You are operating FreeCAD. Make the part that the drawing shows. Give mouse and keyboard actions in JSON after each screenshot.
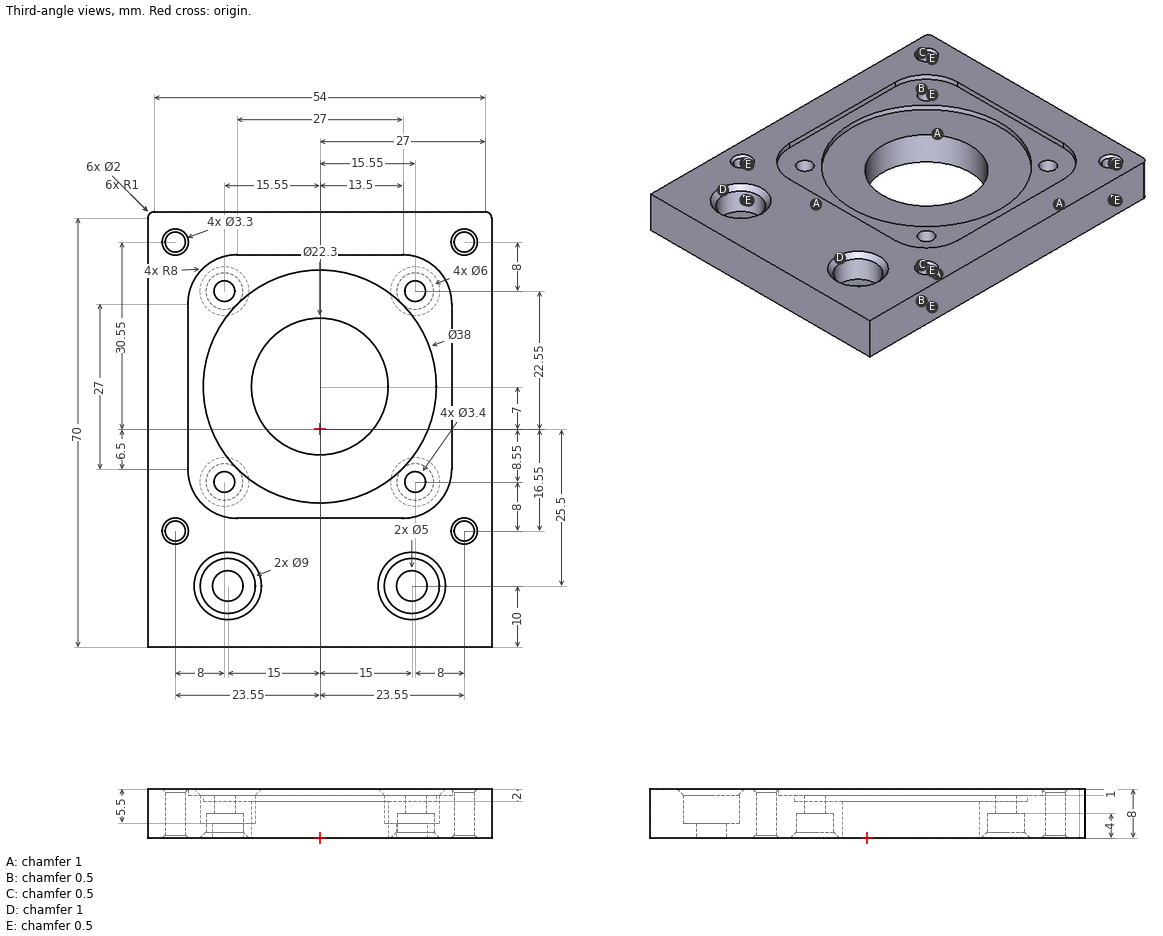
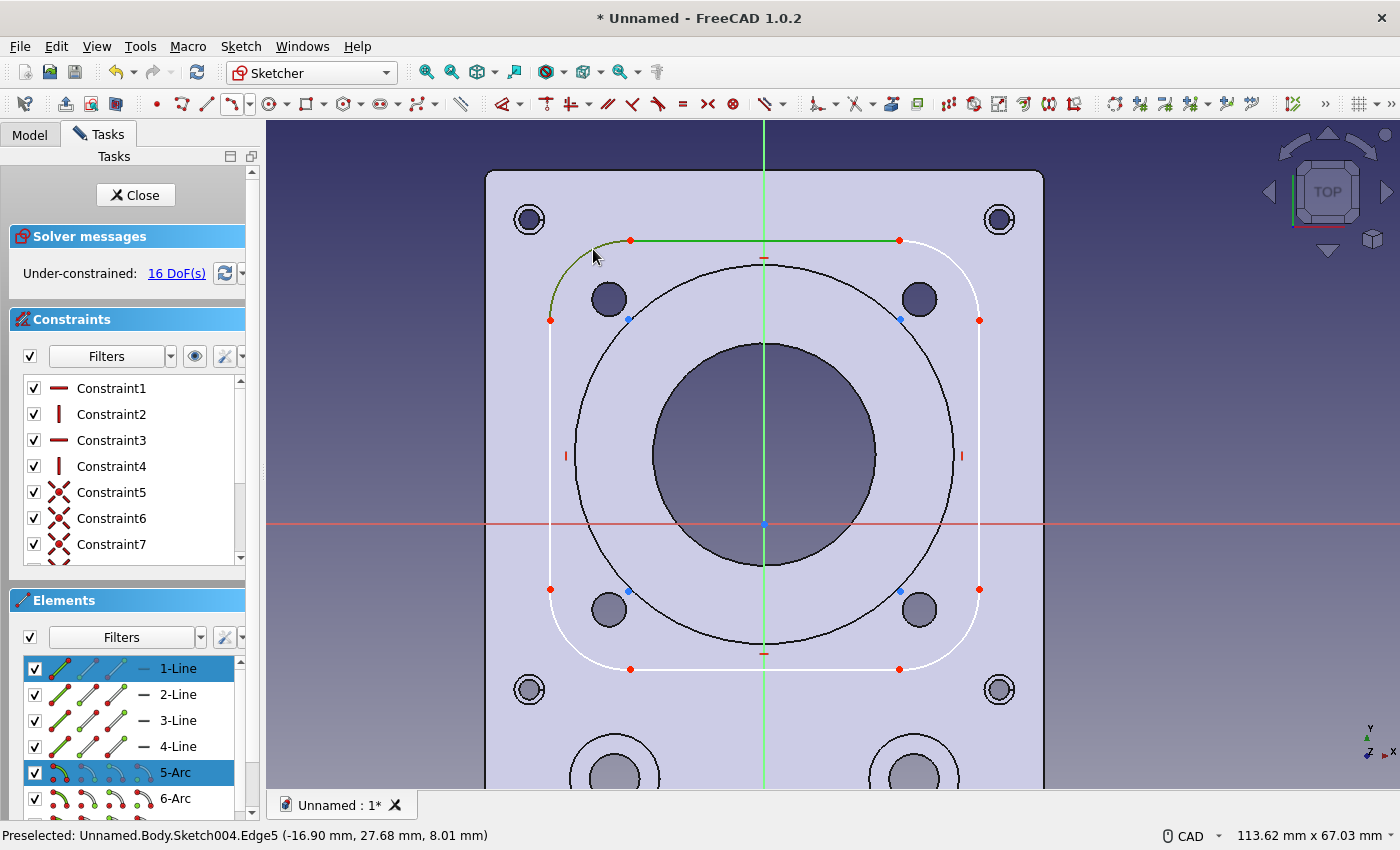
{"action": "key", "text": "t"}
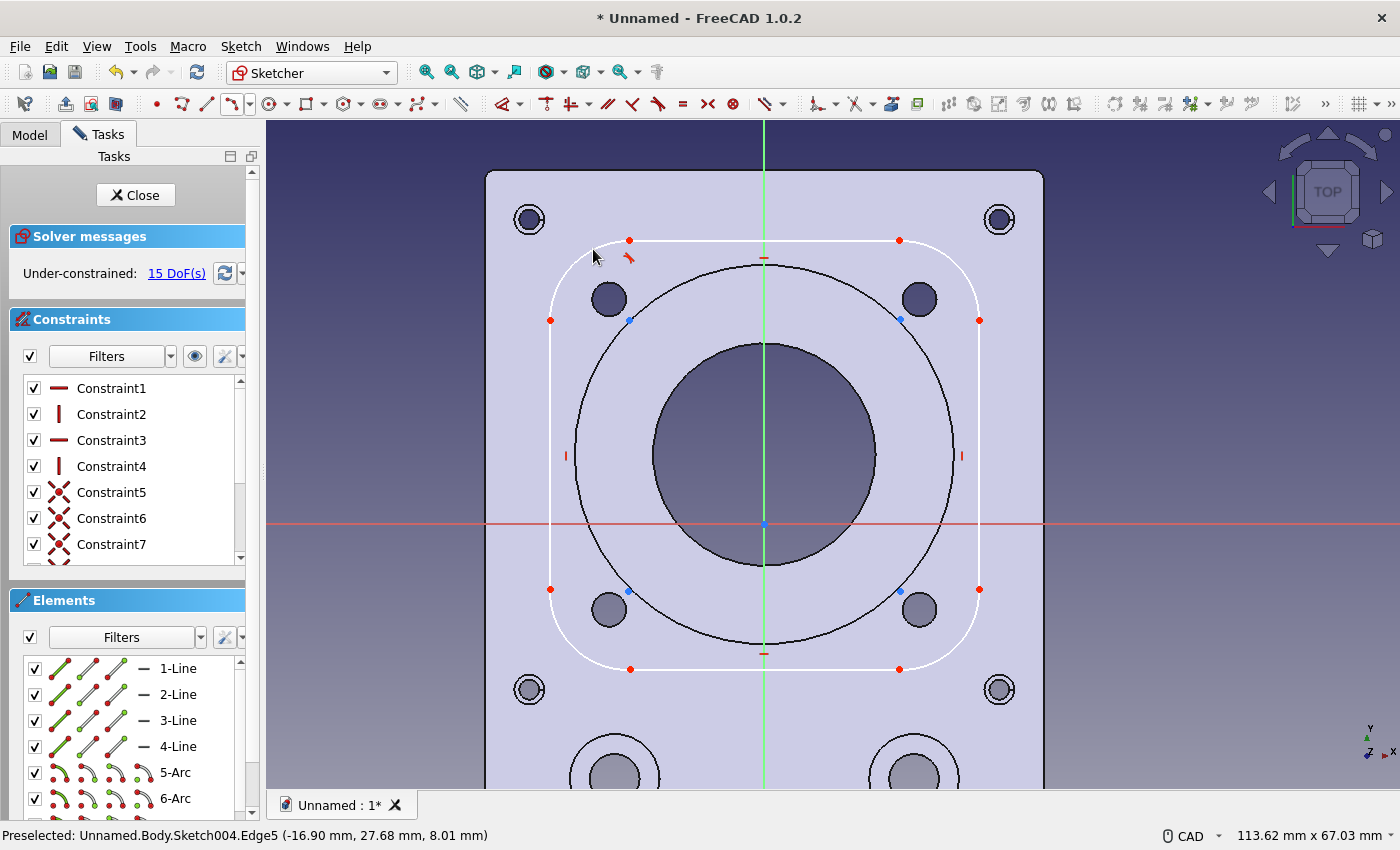
{"action": "left_click", "coordinate": [818, 241]}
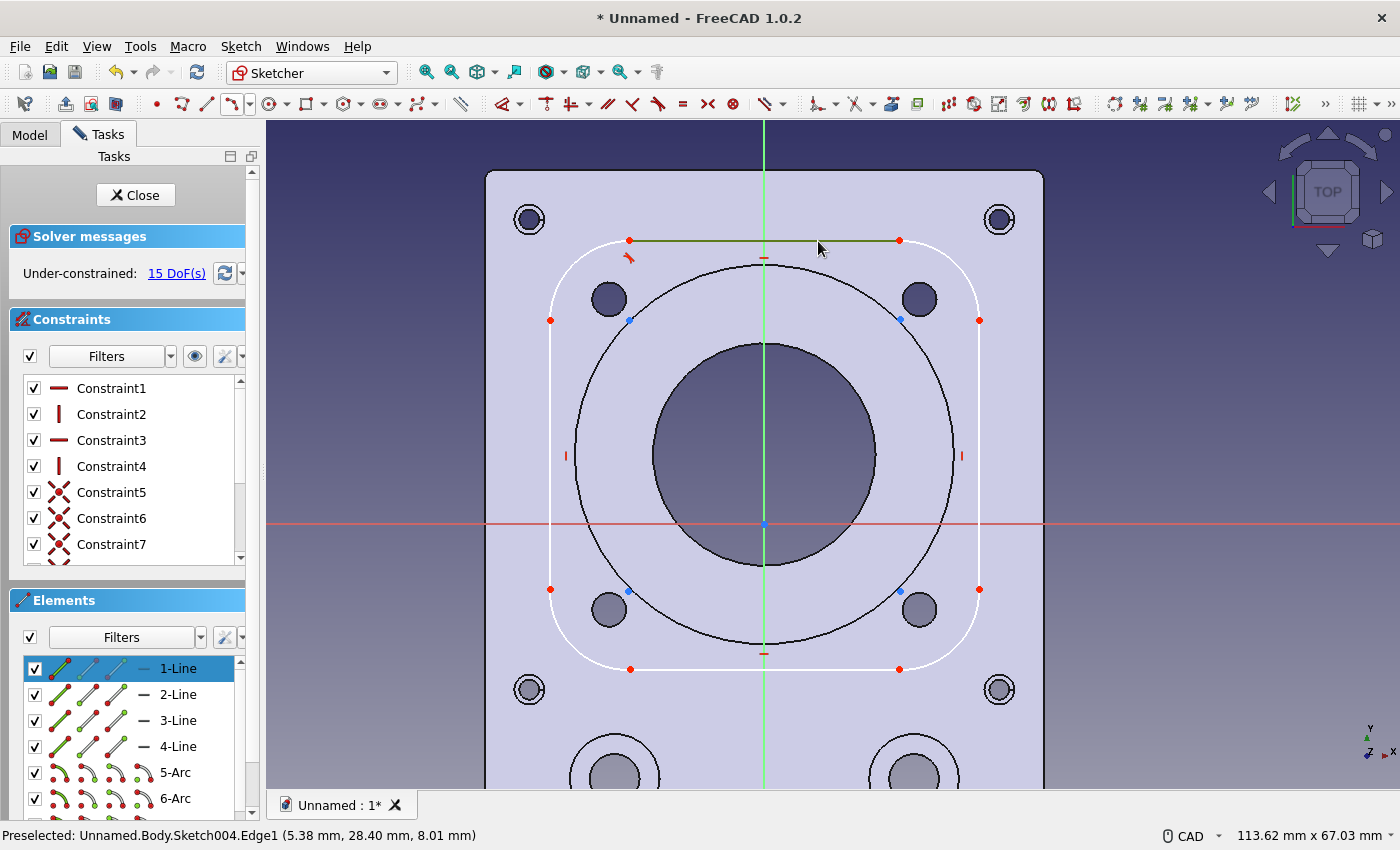
{"action": "left_click", "coordinate": [971, 284]}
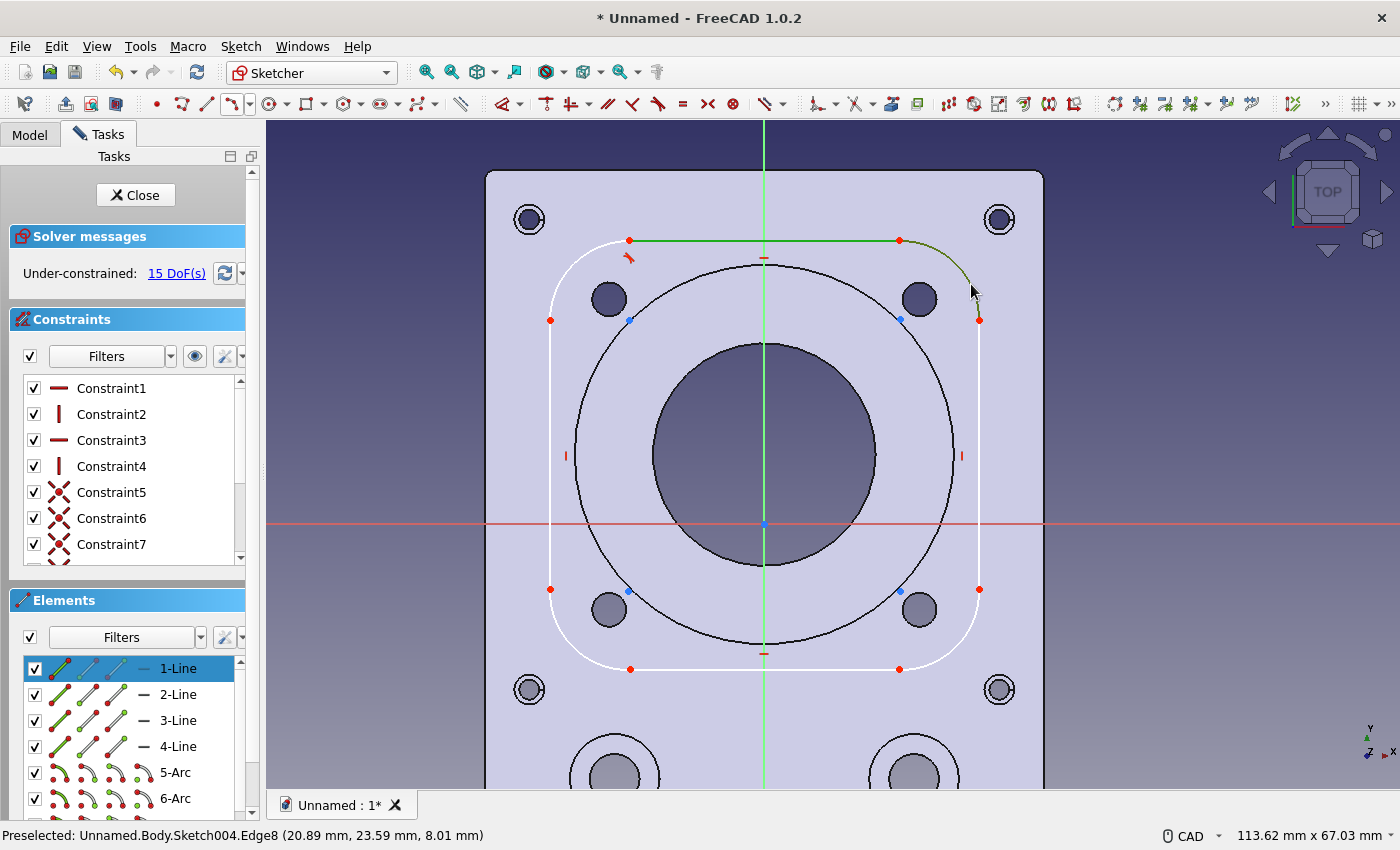
{"action": "key", "text": "t"}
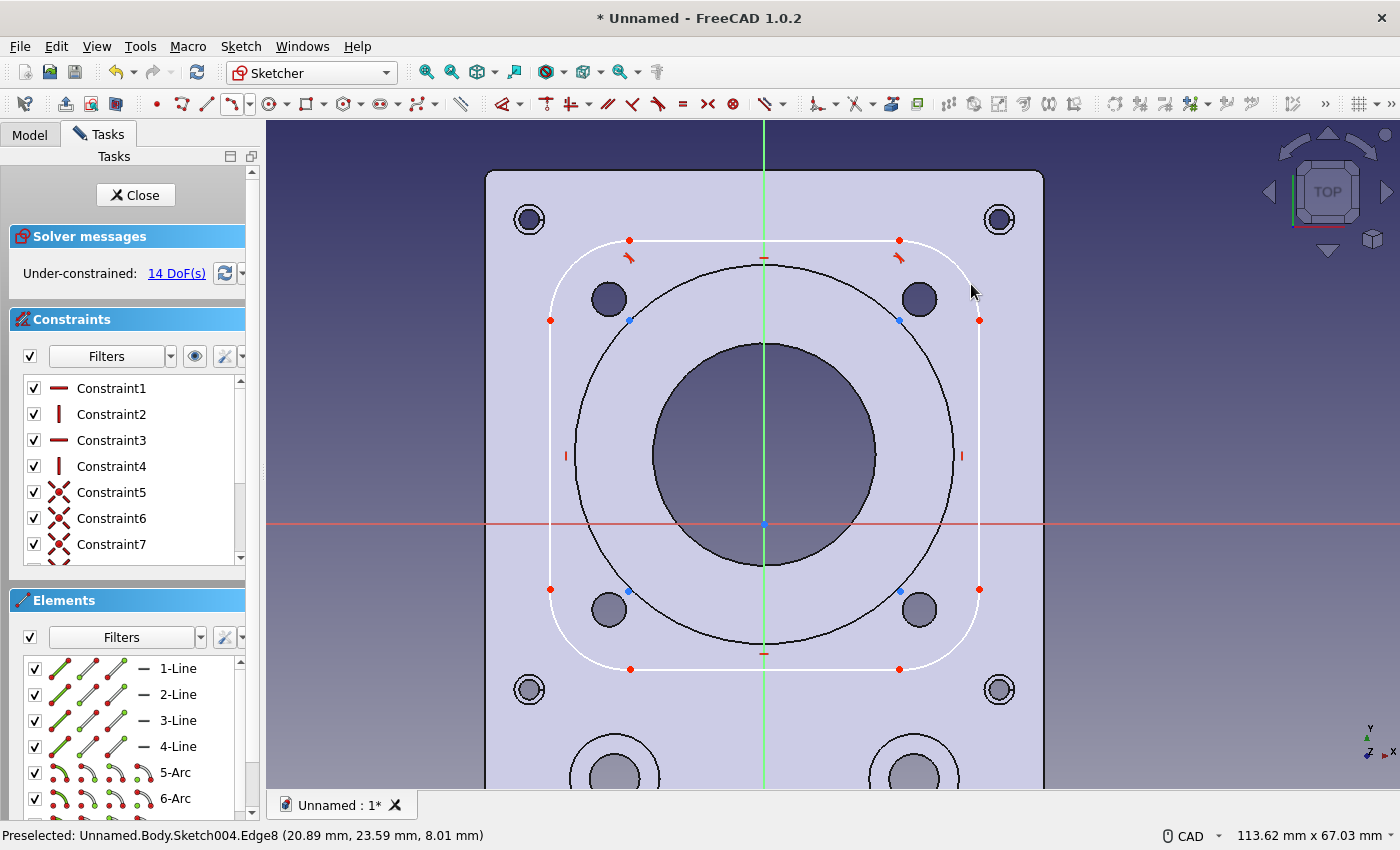
{"action": "left_click", "coordinate": [550, 402]}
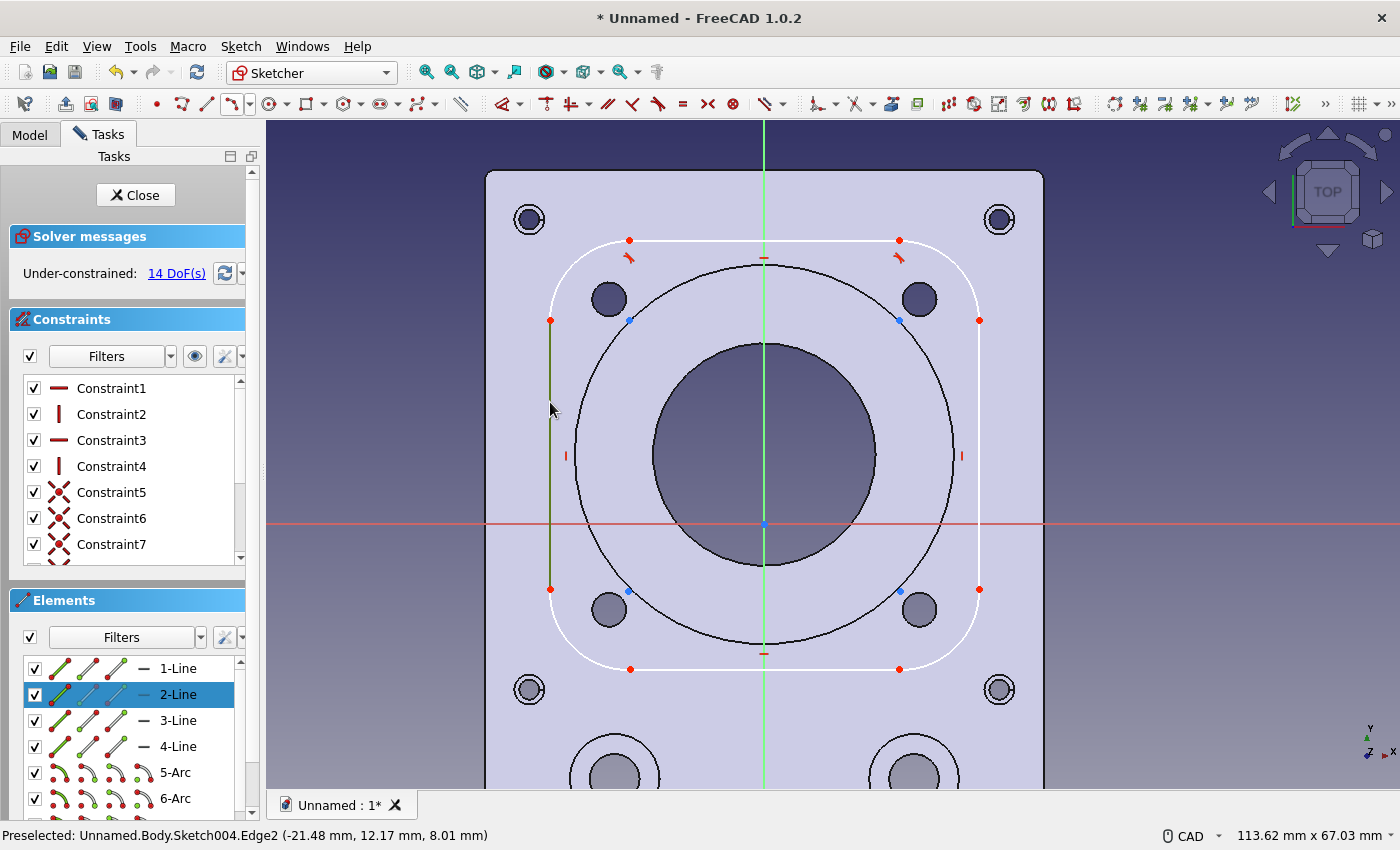
{"action": "left_click", "coordinate": [594, 250]}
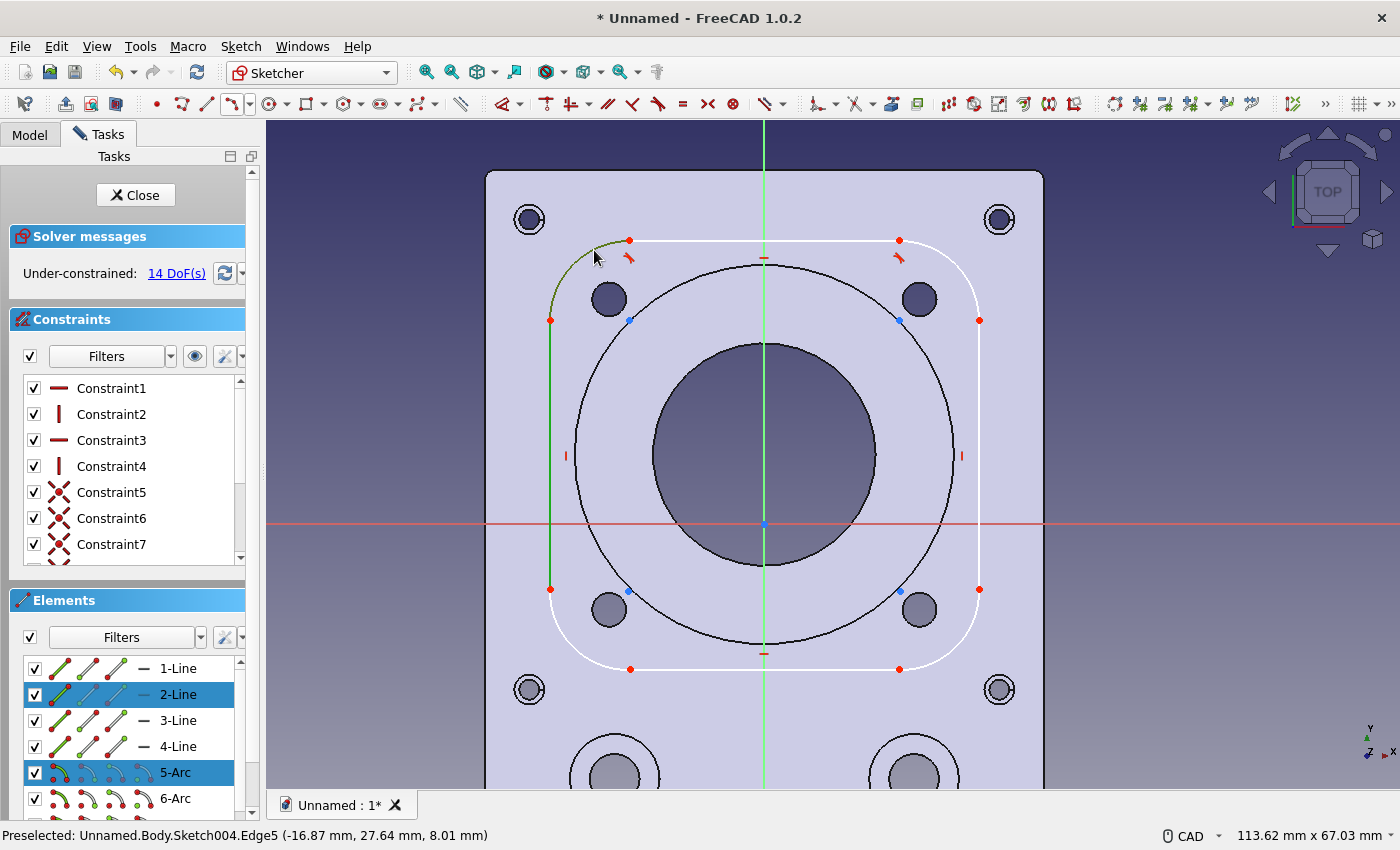
{"action": "key", "text": "t"}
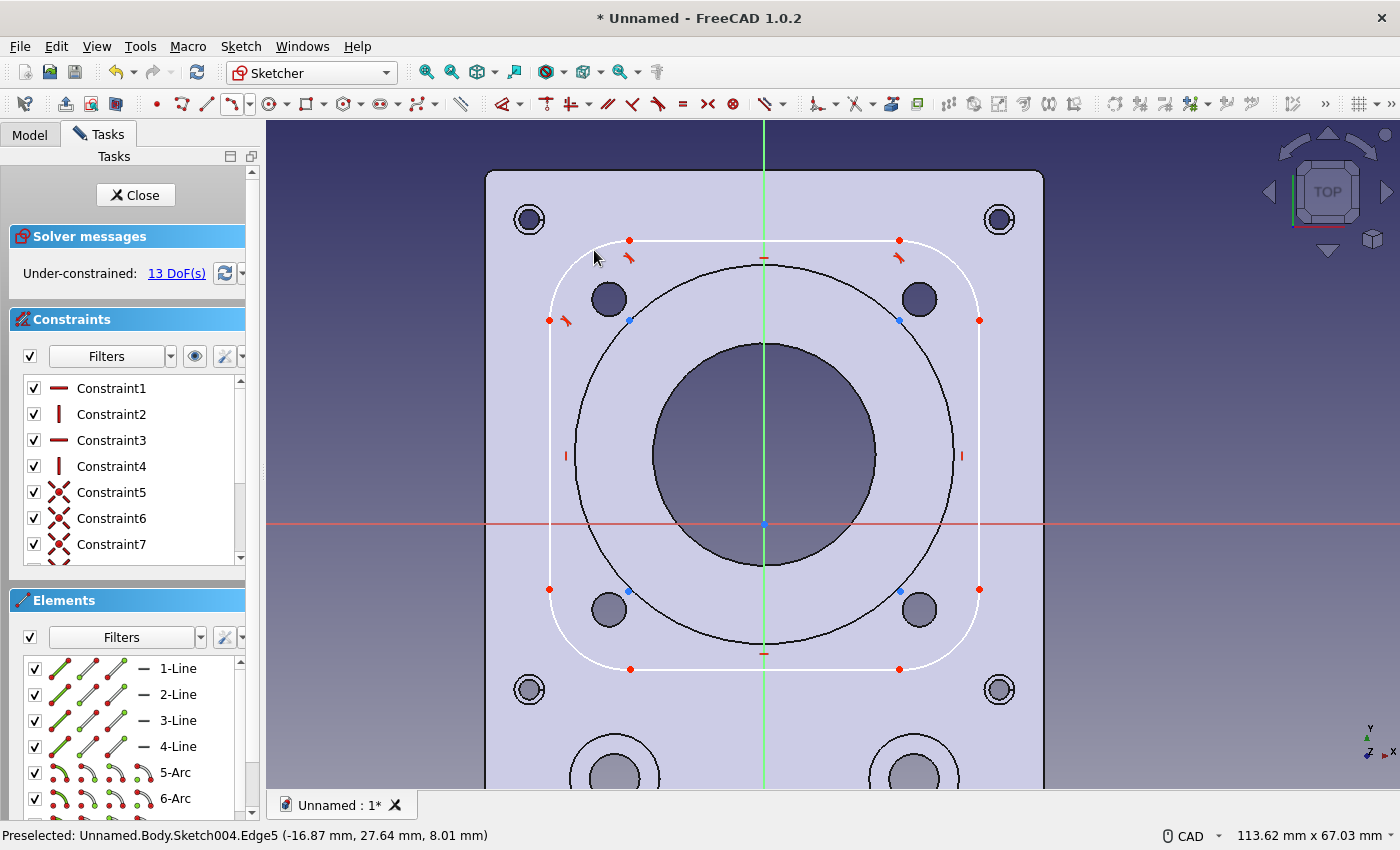
{"action": "left_click", "coordinate": [550, 402]}